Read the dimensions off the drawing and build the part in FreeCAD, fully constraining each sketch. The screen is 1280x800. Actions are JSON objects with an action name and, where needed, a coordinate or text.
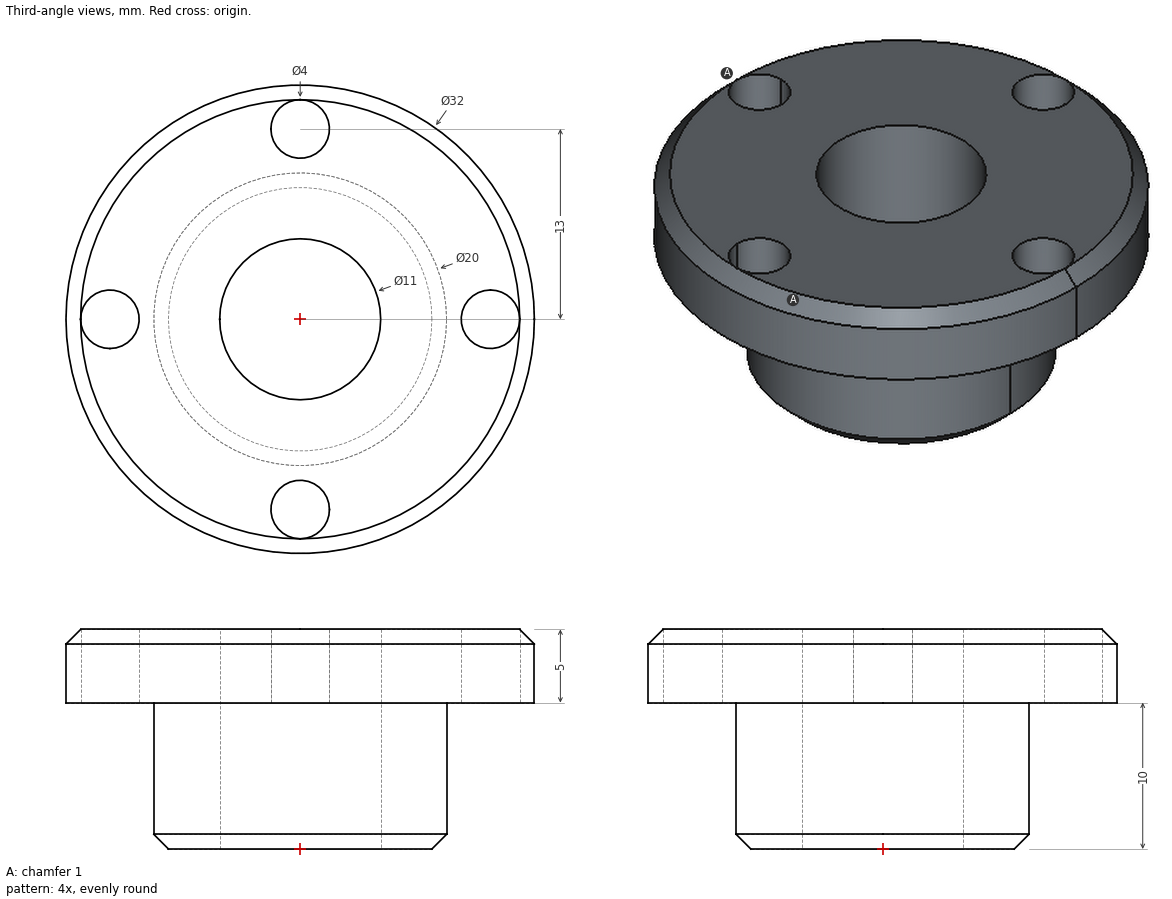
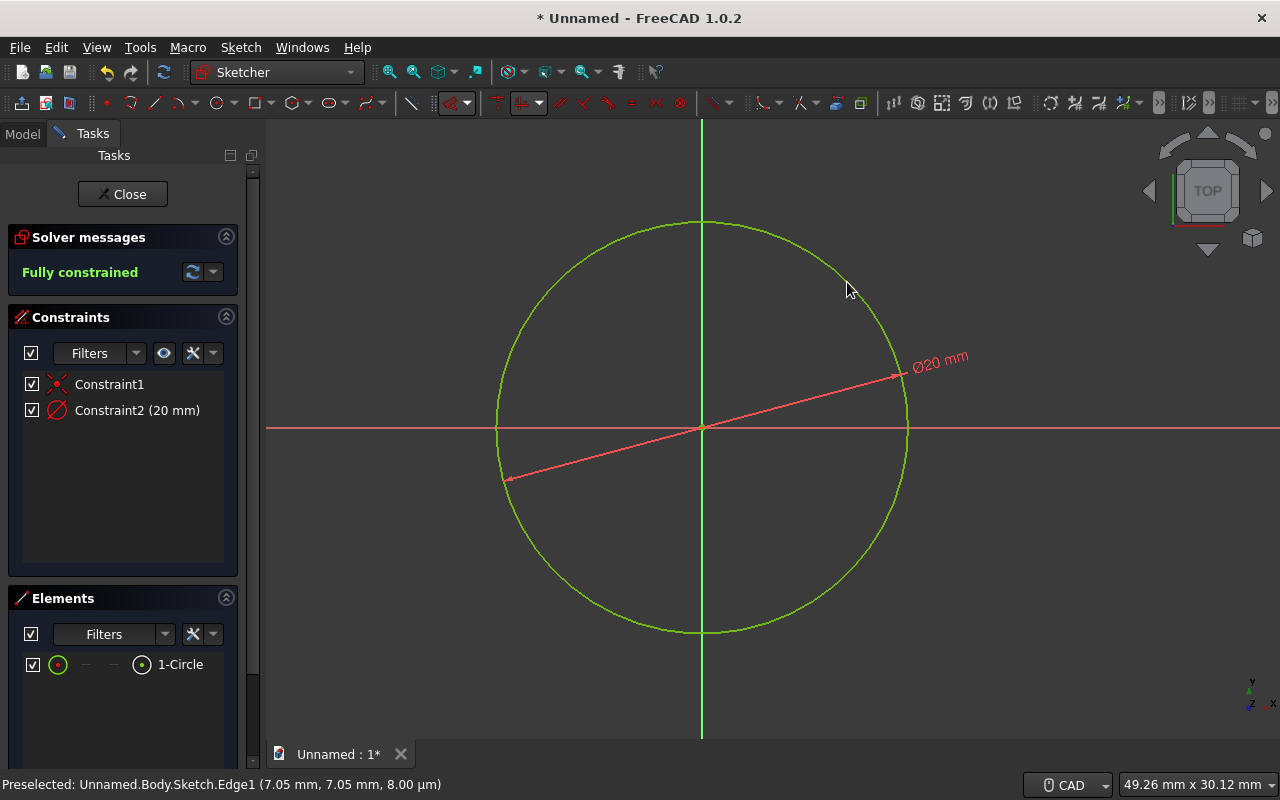
{"action": "left_click", "coordinate": [123, 194]}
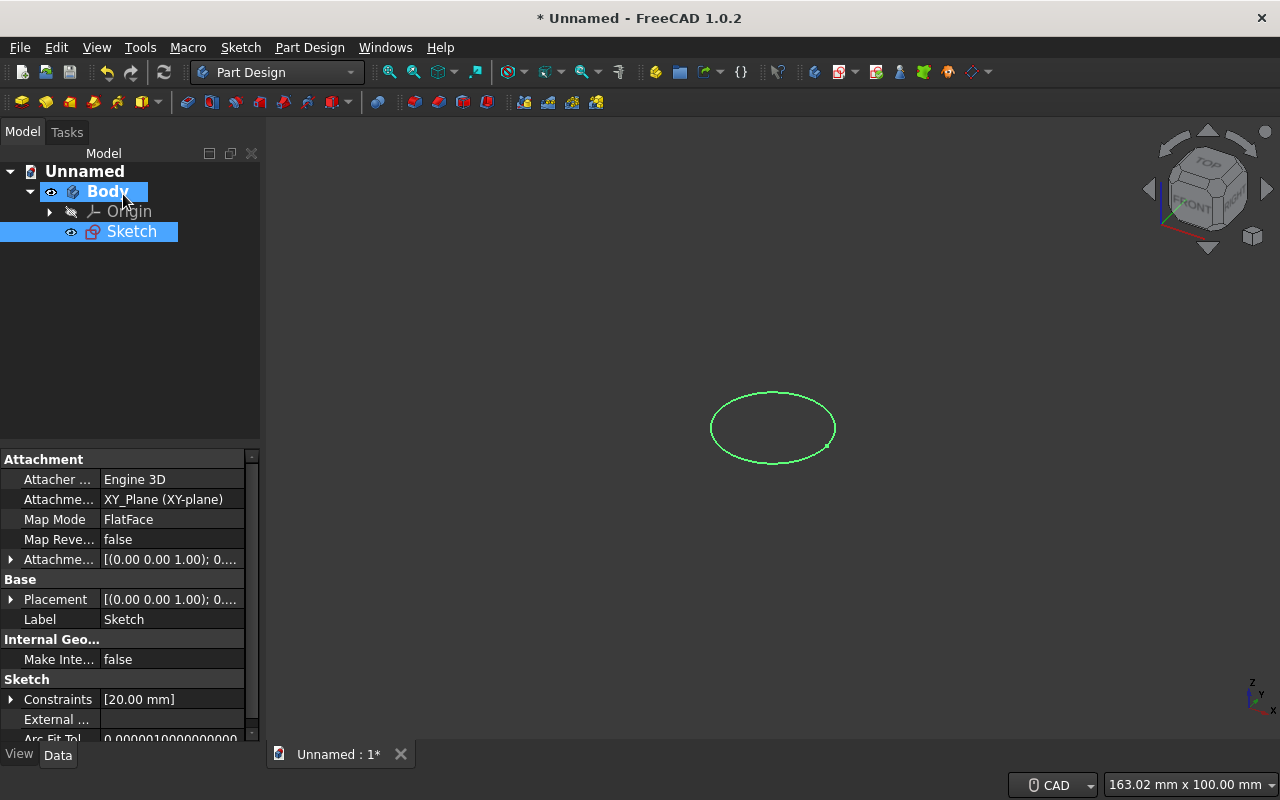
{"action": "left_click", "coordinate": [22, 102]}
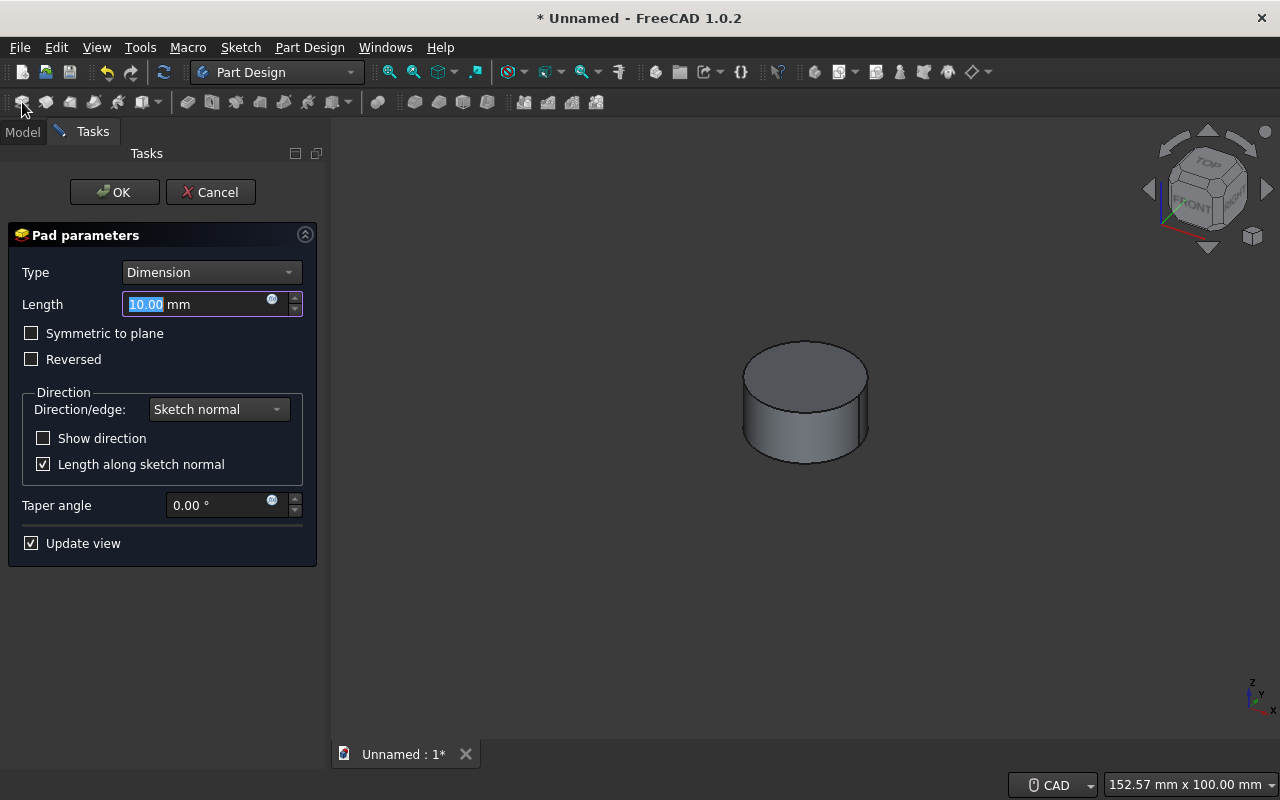
{"action": "type", "text": "10"}
{"action": "key", "text": "Tab"}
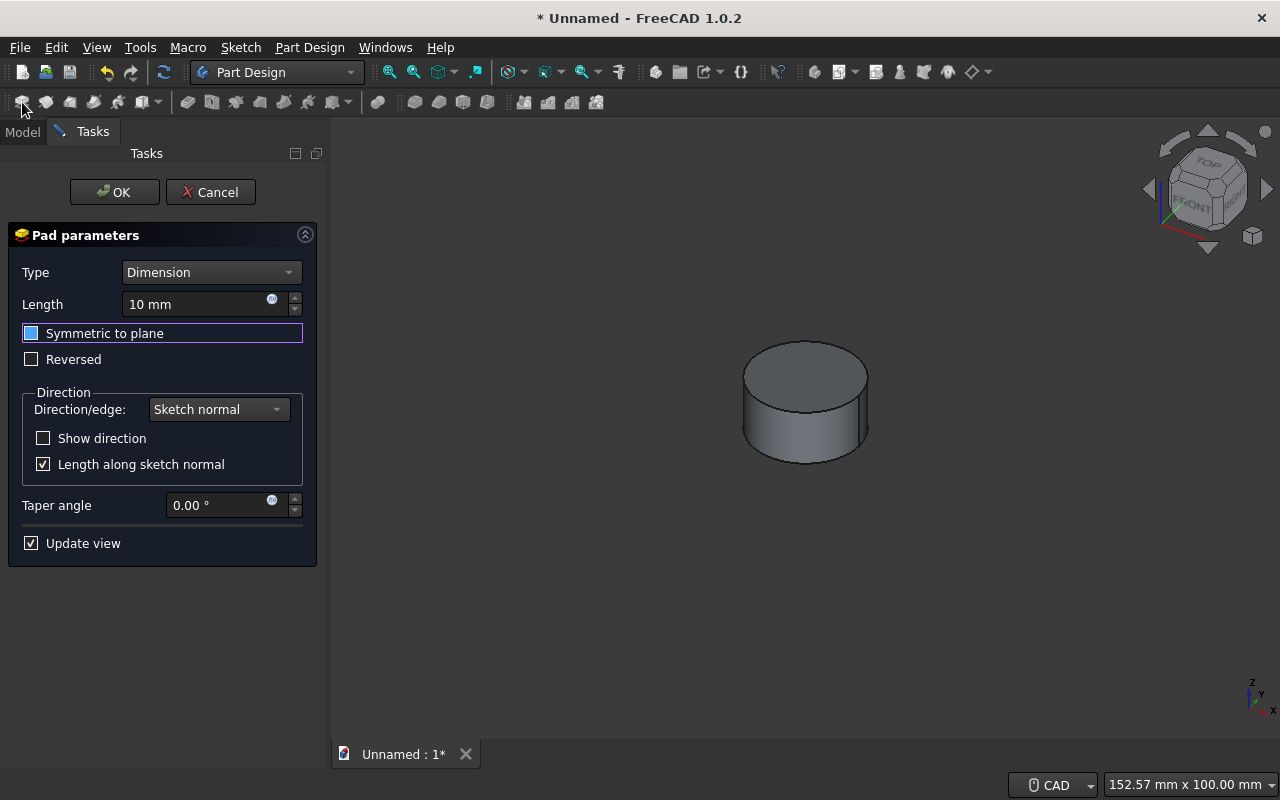
{"action": "left_click", "coordinate": [115, 192]}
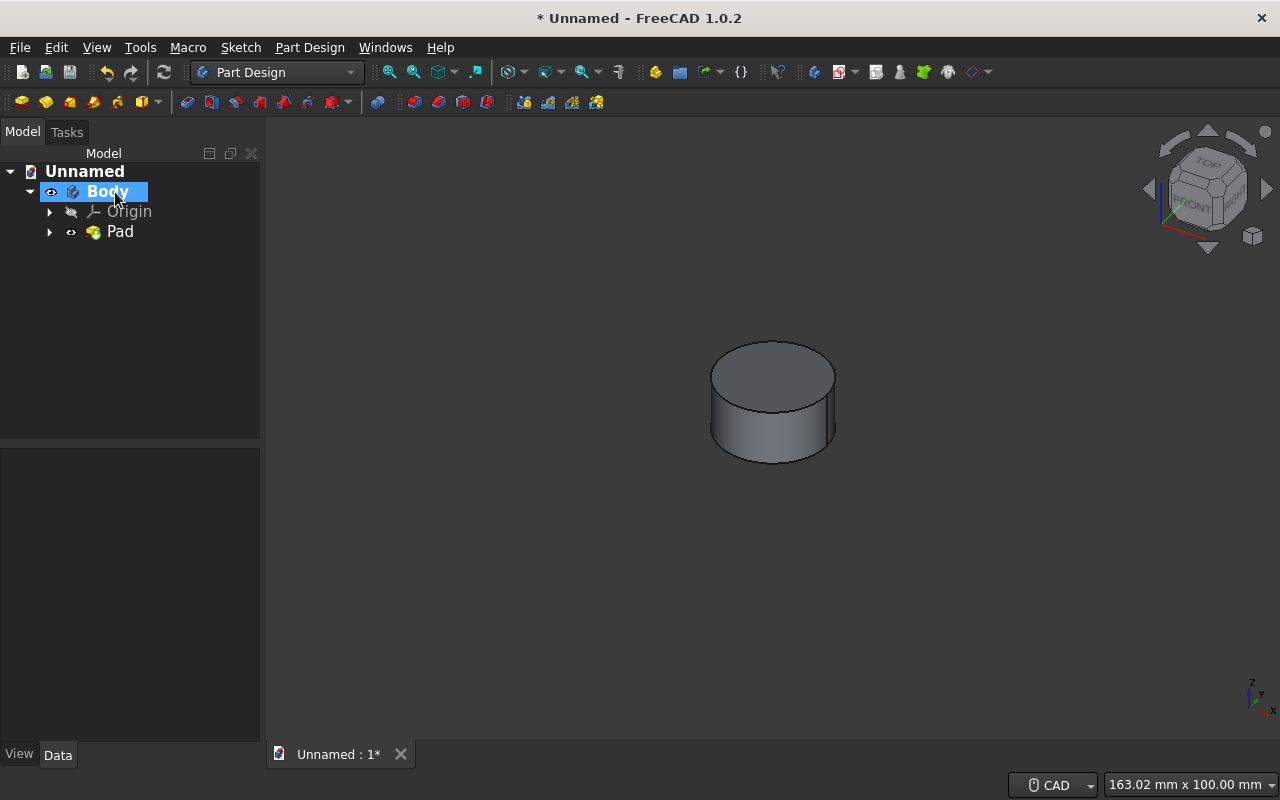
{"action": "key", "text": "v f"}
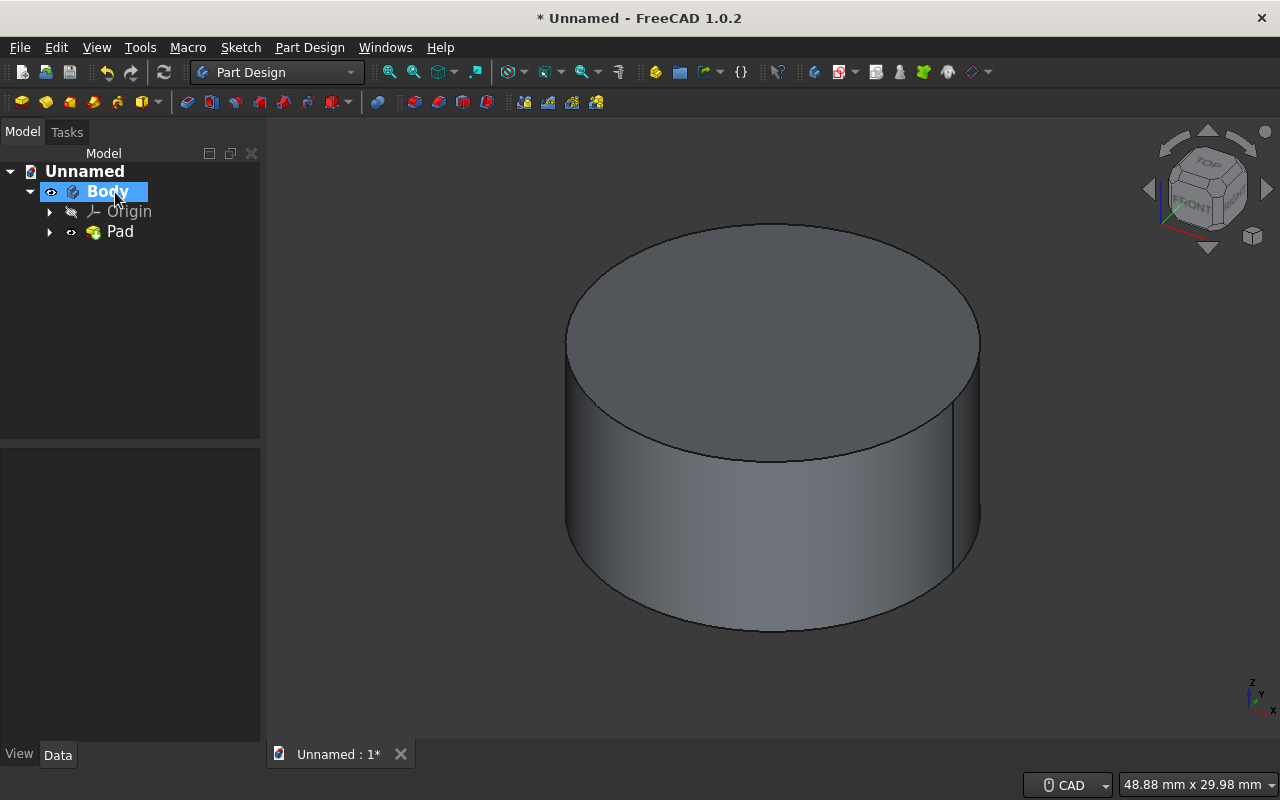
{"action": "left_click", "coordinate": [773, 342]}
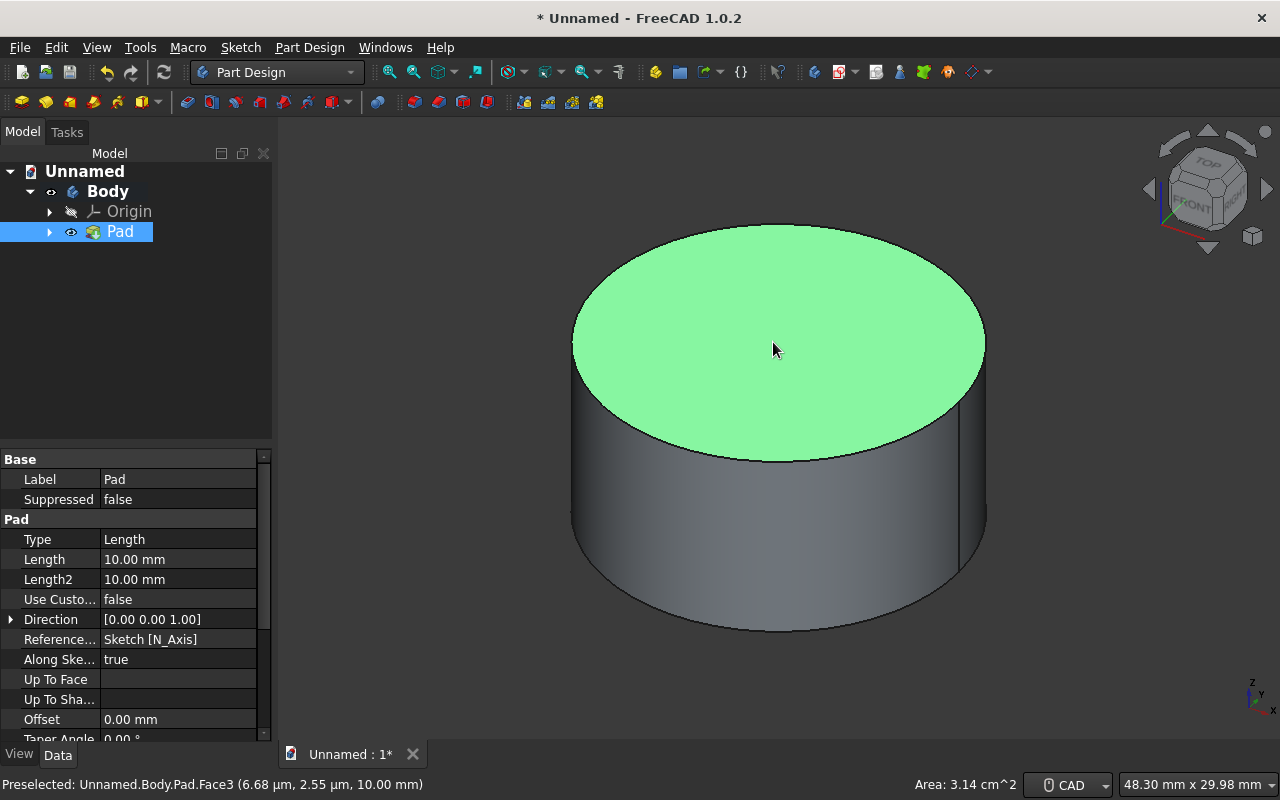
{"action": "left_click", "coordinate": [840, 72]}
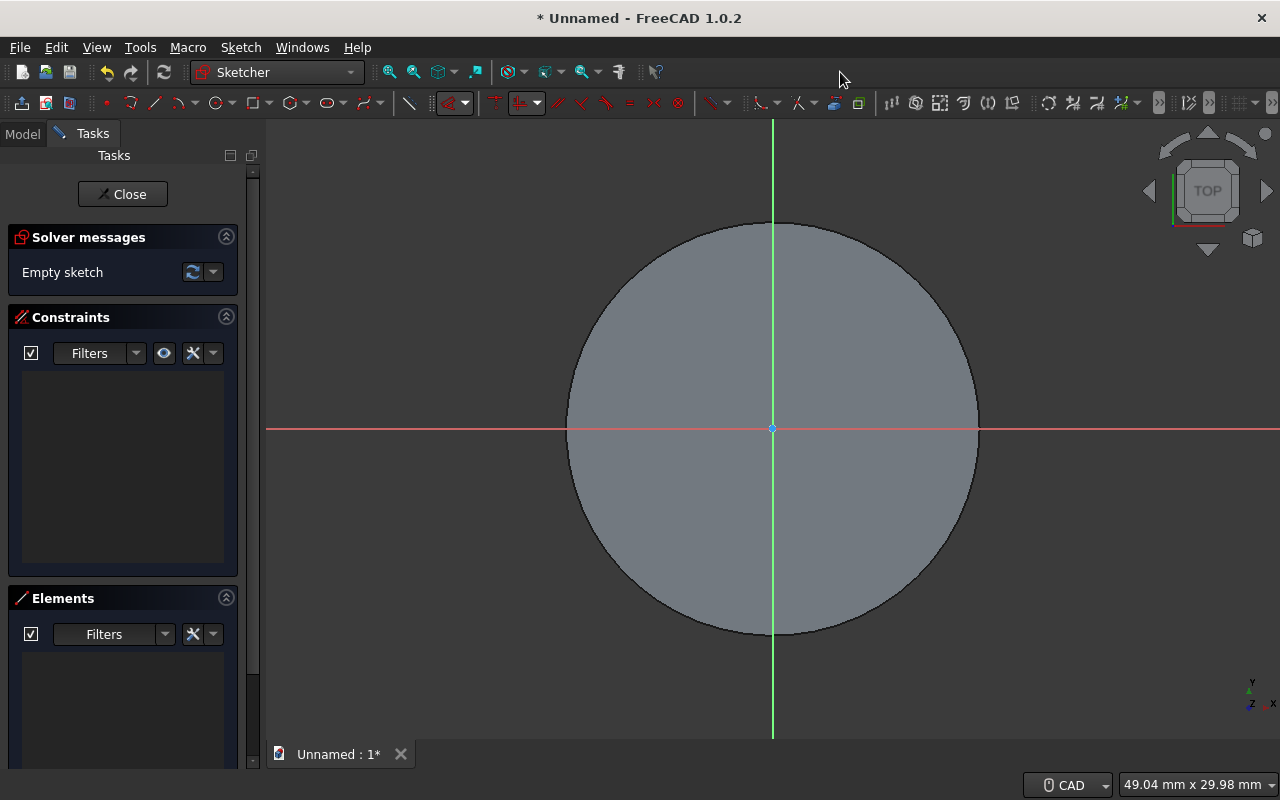
{"action": "scroll", "coordinate": [621, 429], "scroll_direction": "down", "scroll_amount": 3}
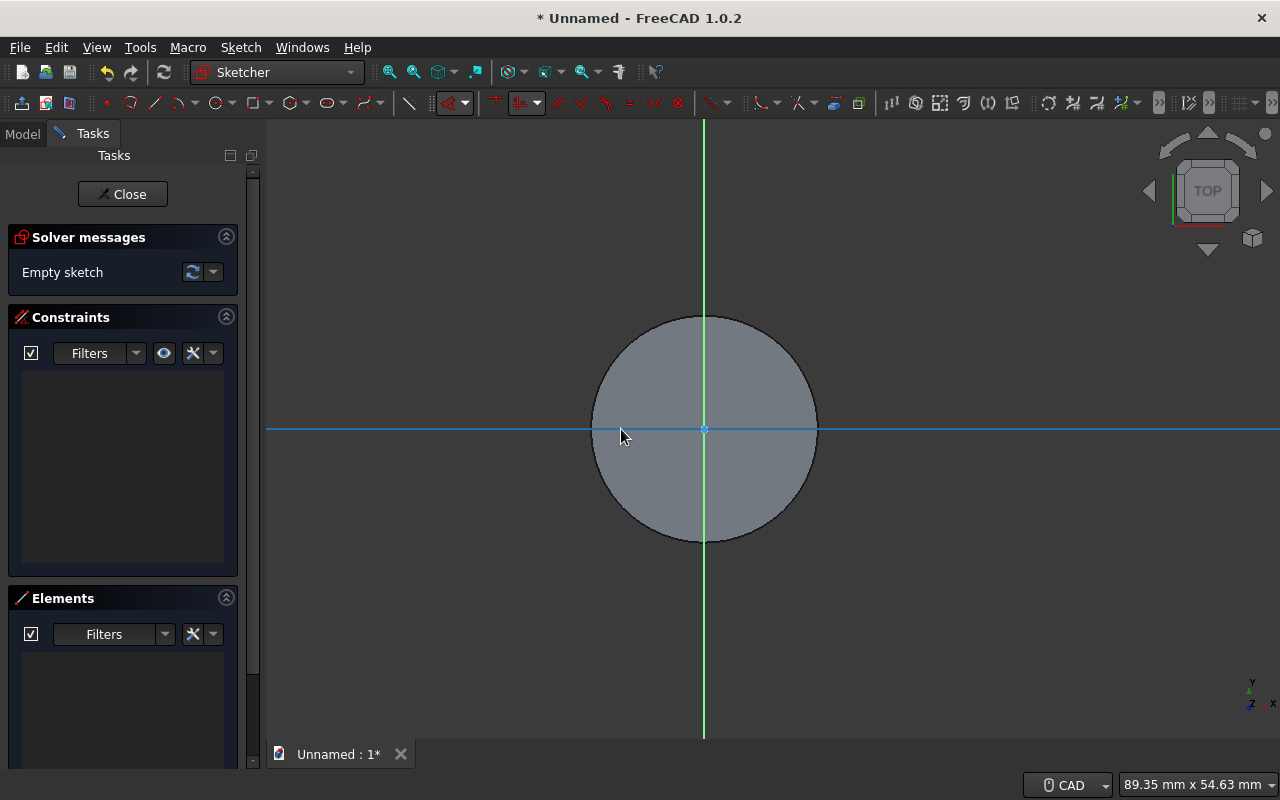
{"action": "left_click", "coordinate": [216, 104]}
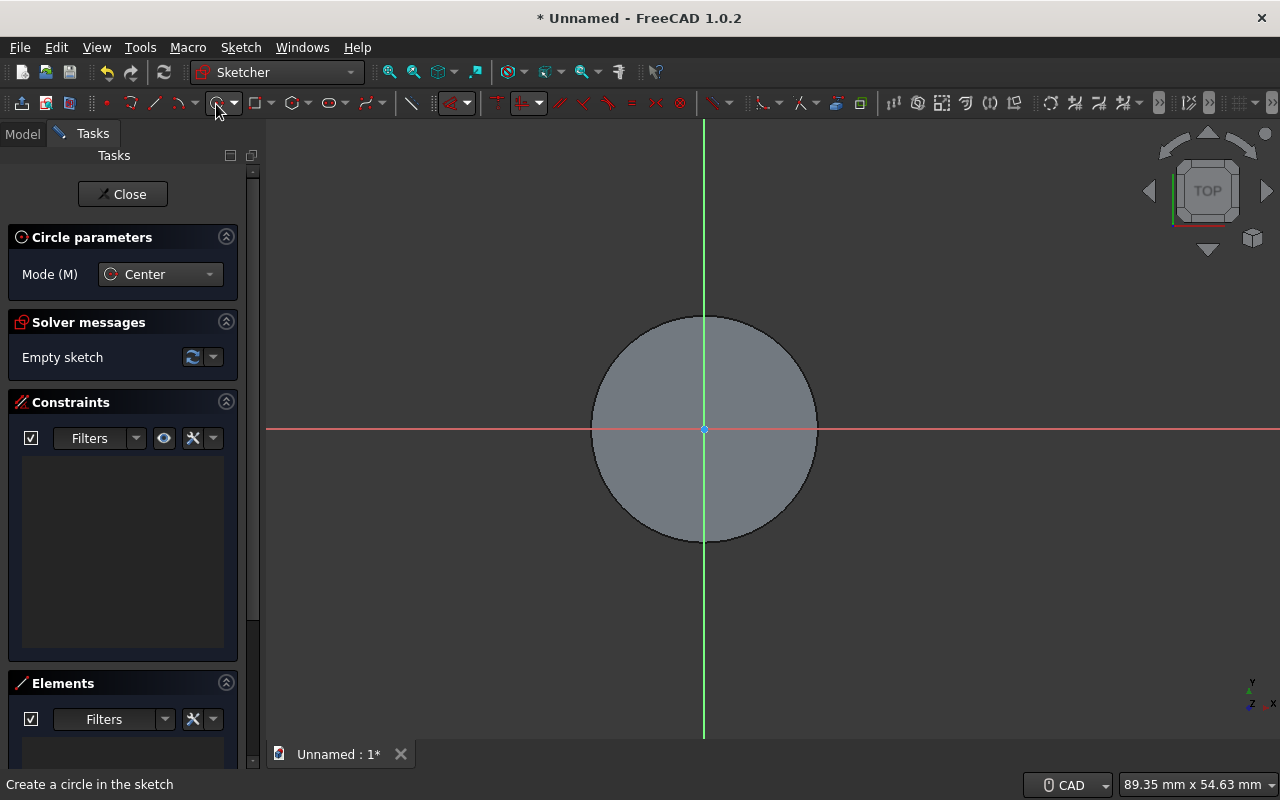
{"action": "left_click", "coordinate": [704, 429]}
{"action": "left_click", "coordinate": [833, 301]}
{"action": "key", "text": "Escape"}